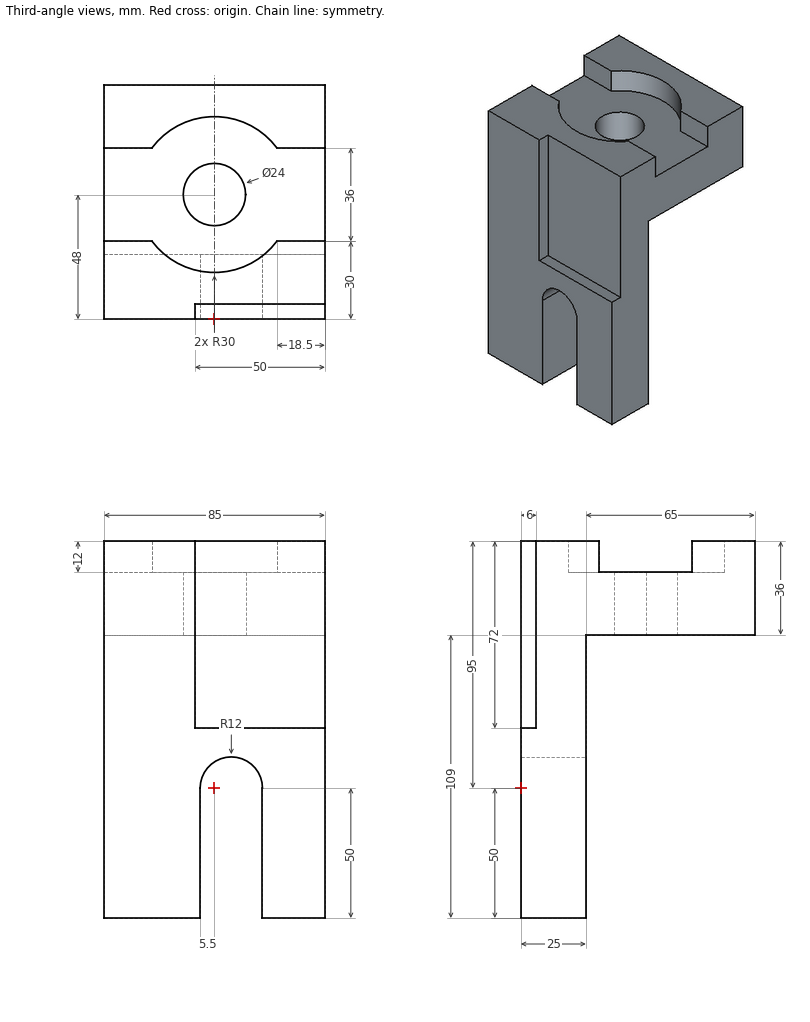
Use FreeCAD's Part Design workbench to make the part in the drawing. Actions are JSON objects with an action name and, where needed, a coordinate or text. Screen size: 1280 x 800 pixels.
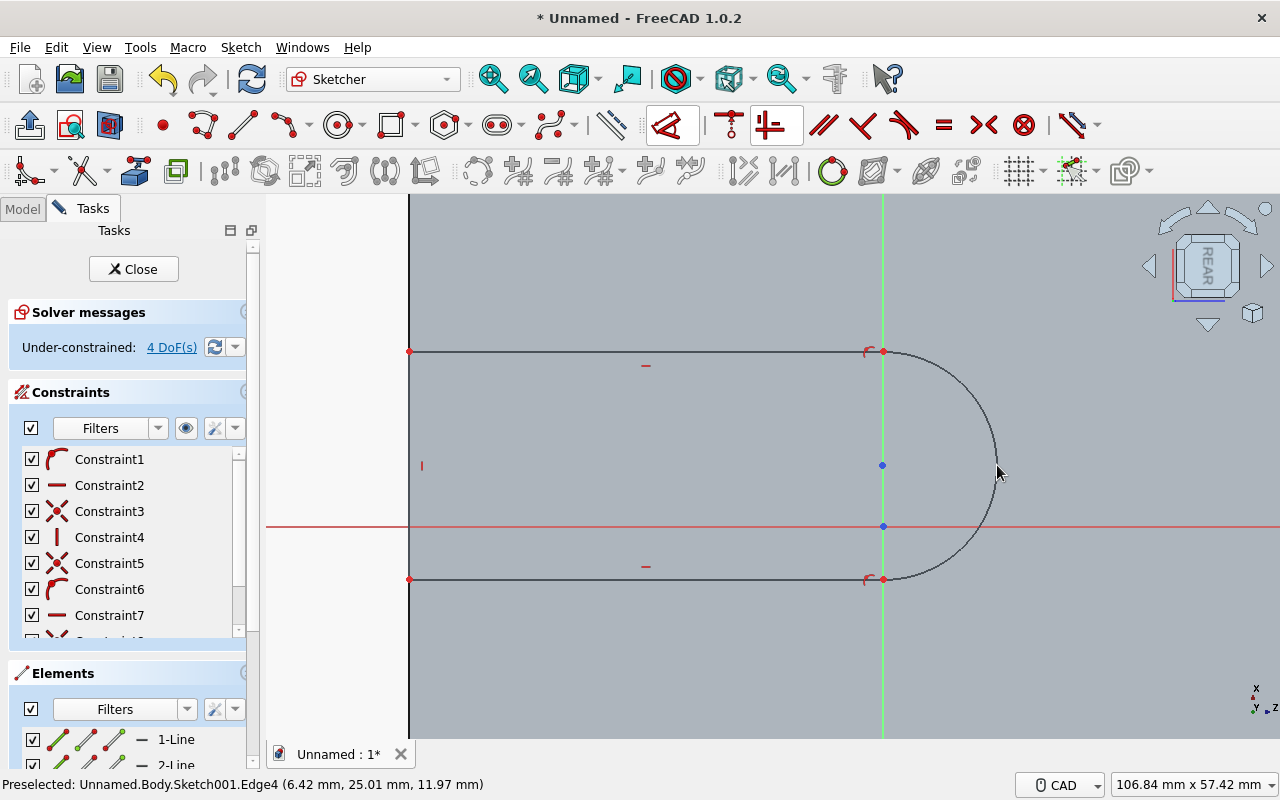
{"action": "left_click", "coordinate": [741, 352]}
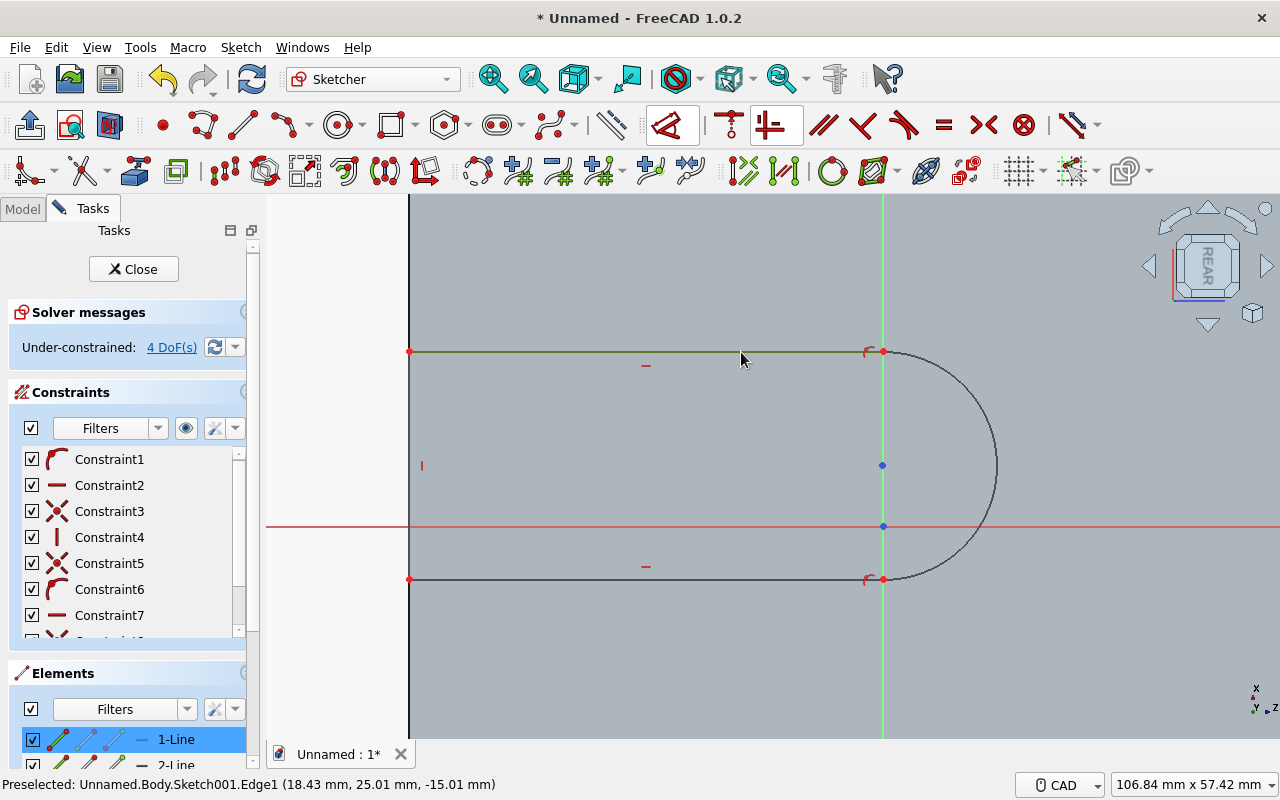
{"action": "left_click", "coordinate": [975, 399]}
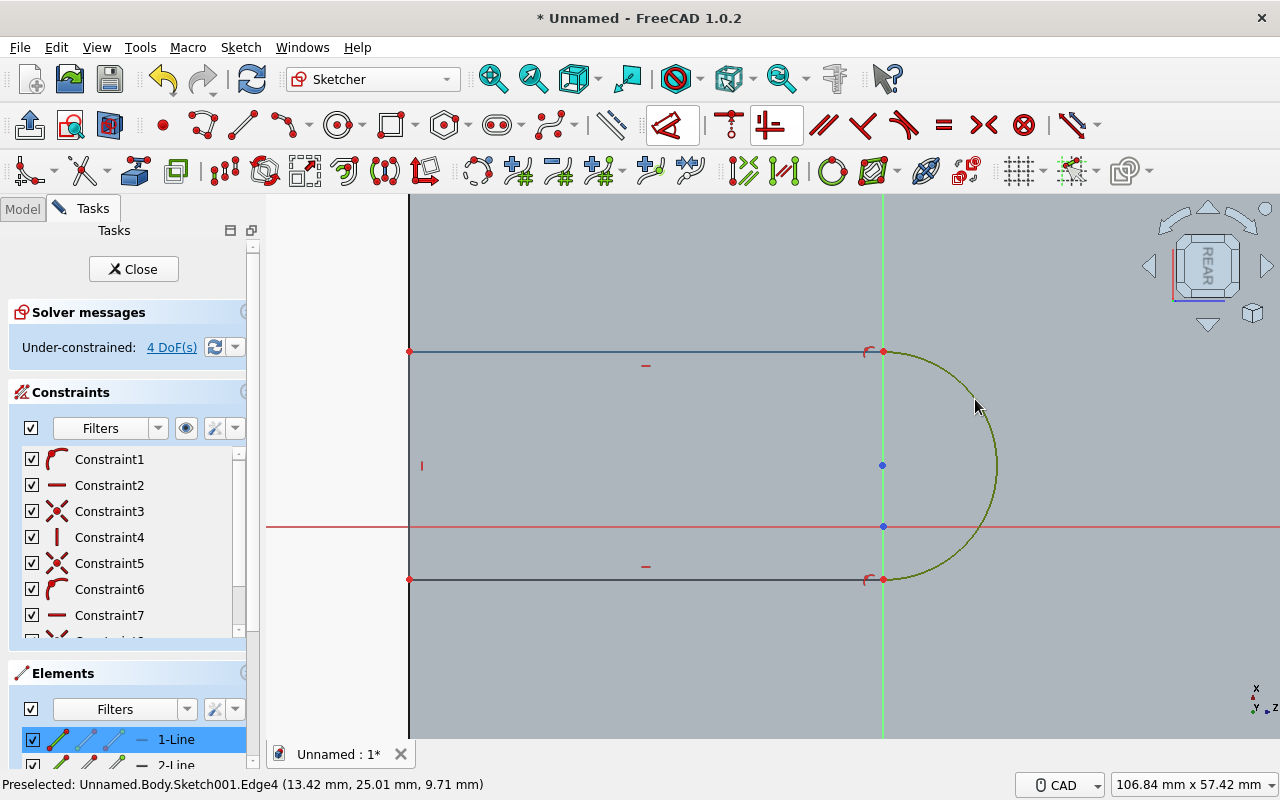
{"action": "left_click", "coordinate": [904, 126]}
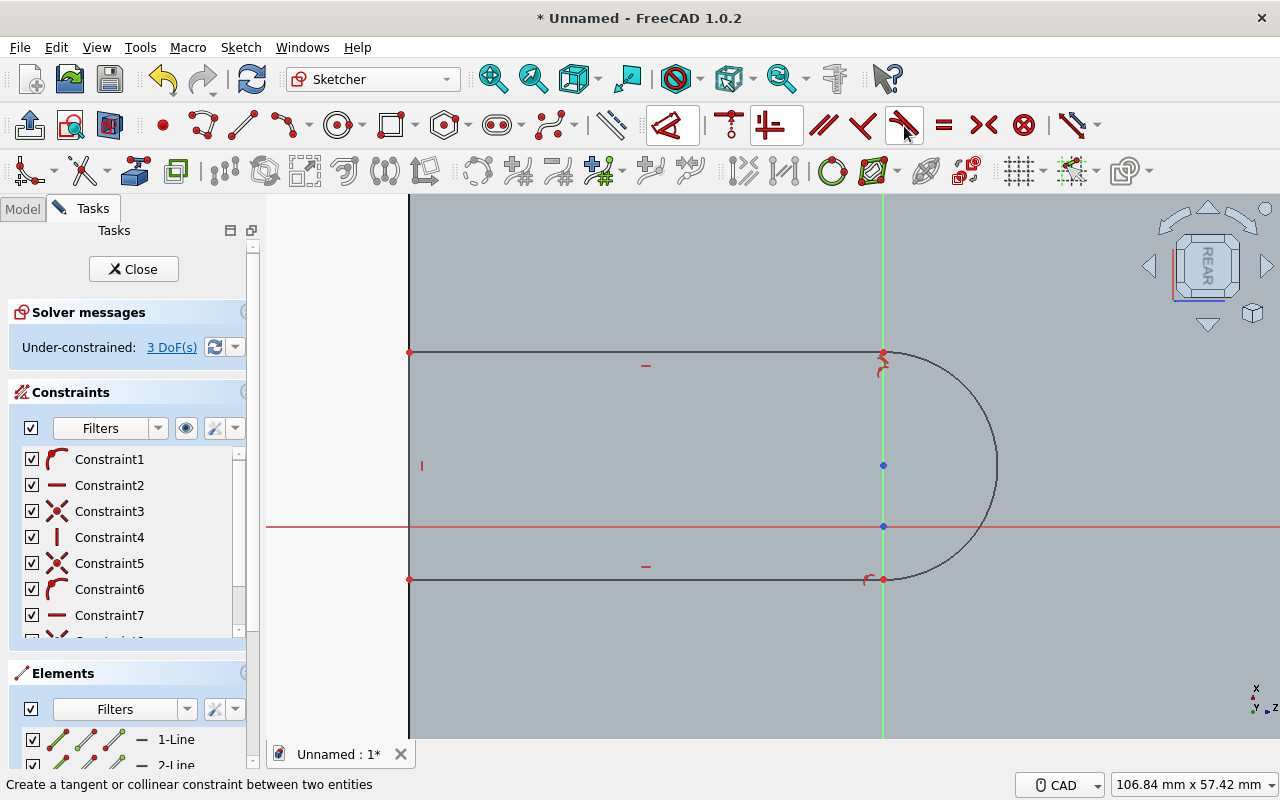
{"action": "left_click", "coordinate": [976, 399]}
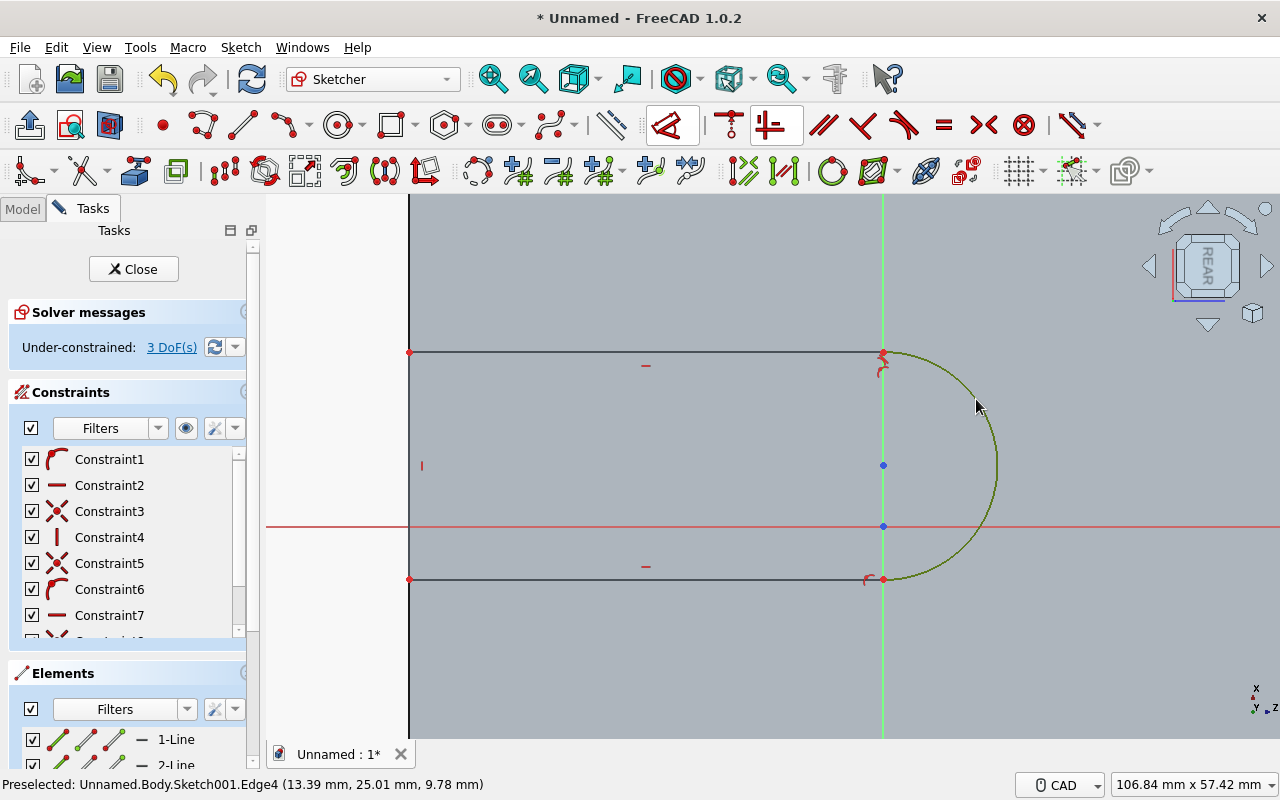
{"action": "left_click", "coordinate": [694, 126]}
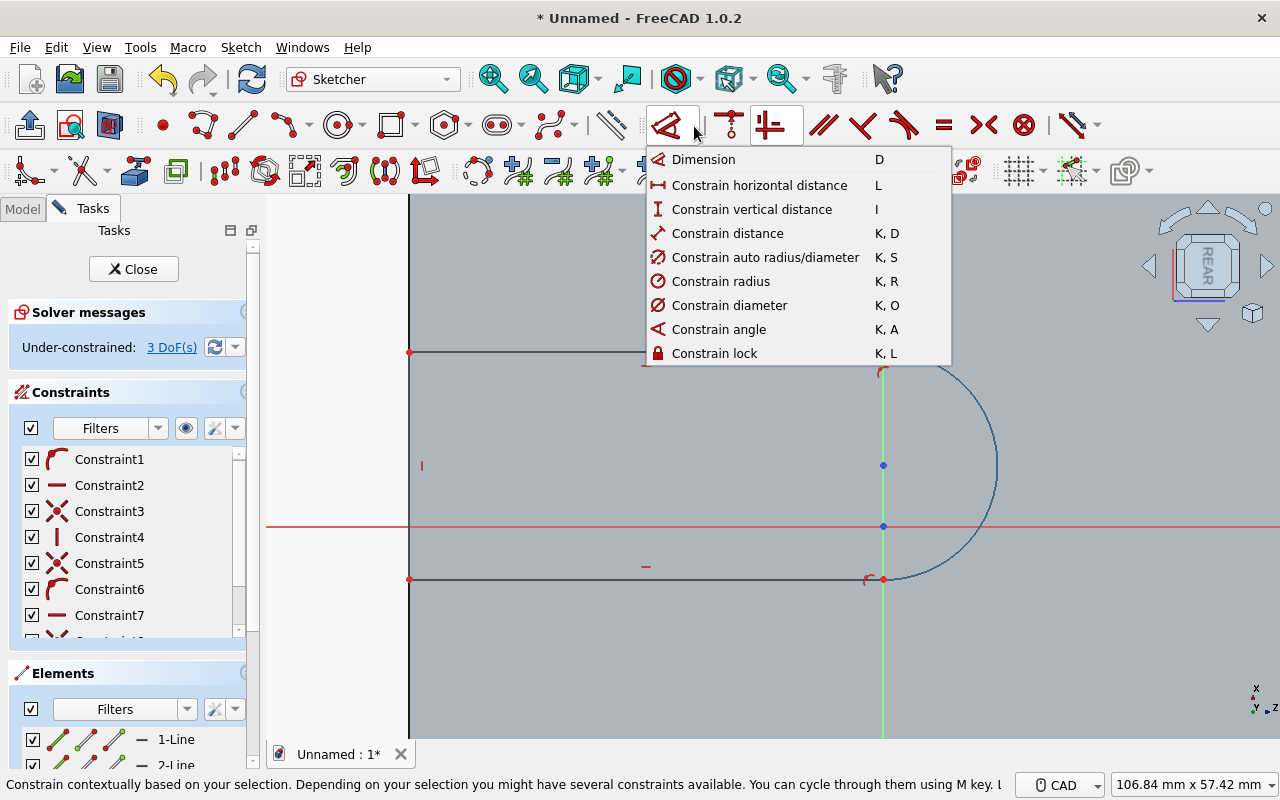
{"action": "left_click", "coordinate": [799, 281]}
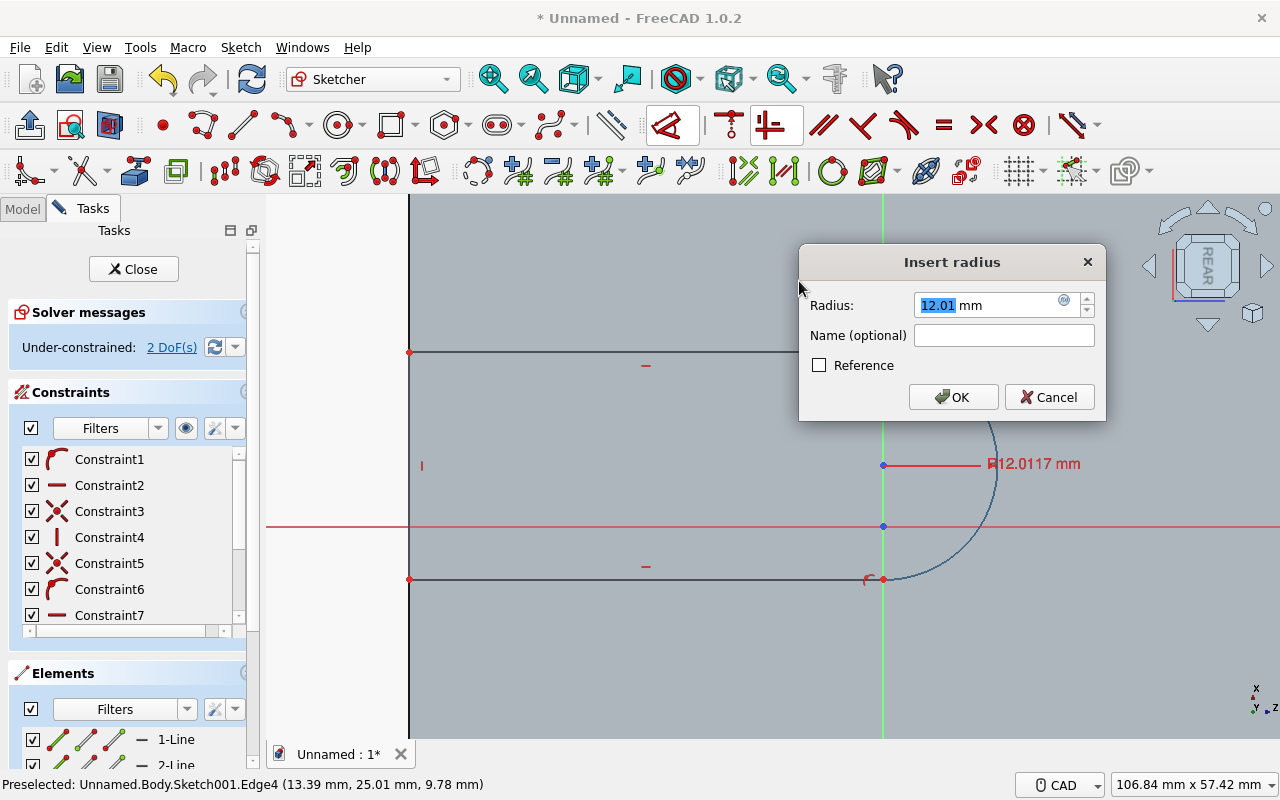
{"action": "type", "text": "12"}
{"action": "key", "text": "Return"}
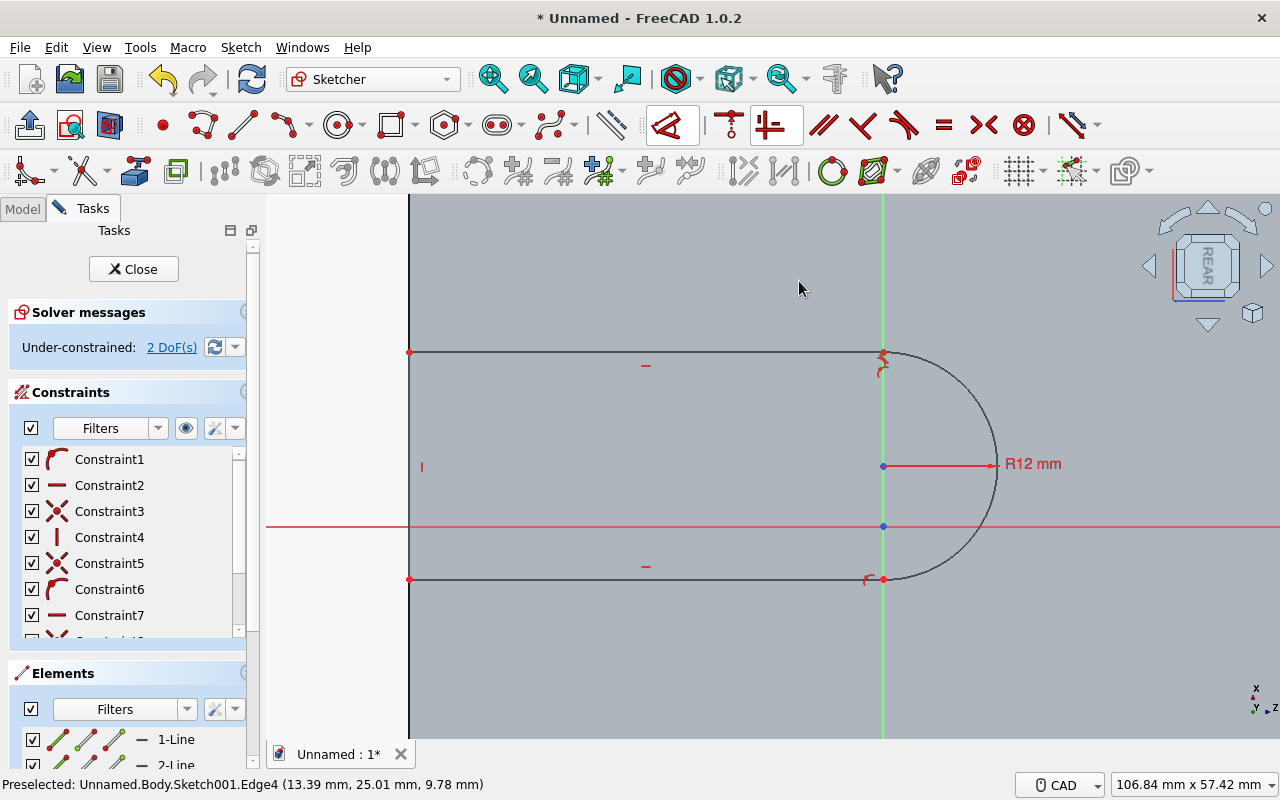
{"action": "left_click", "coordinate": [741, 352]}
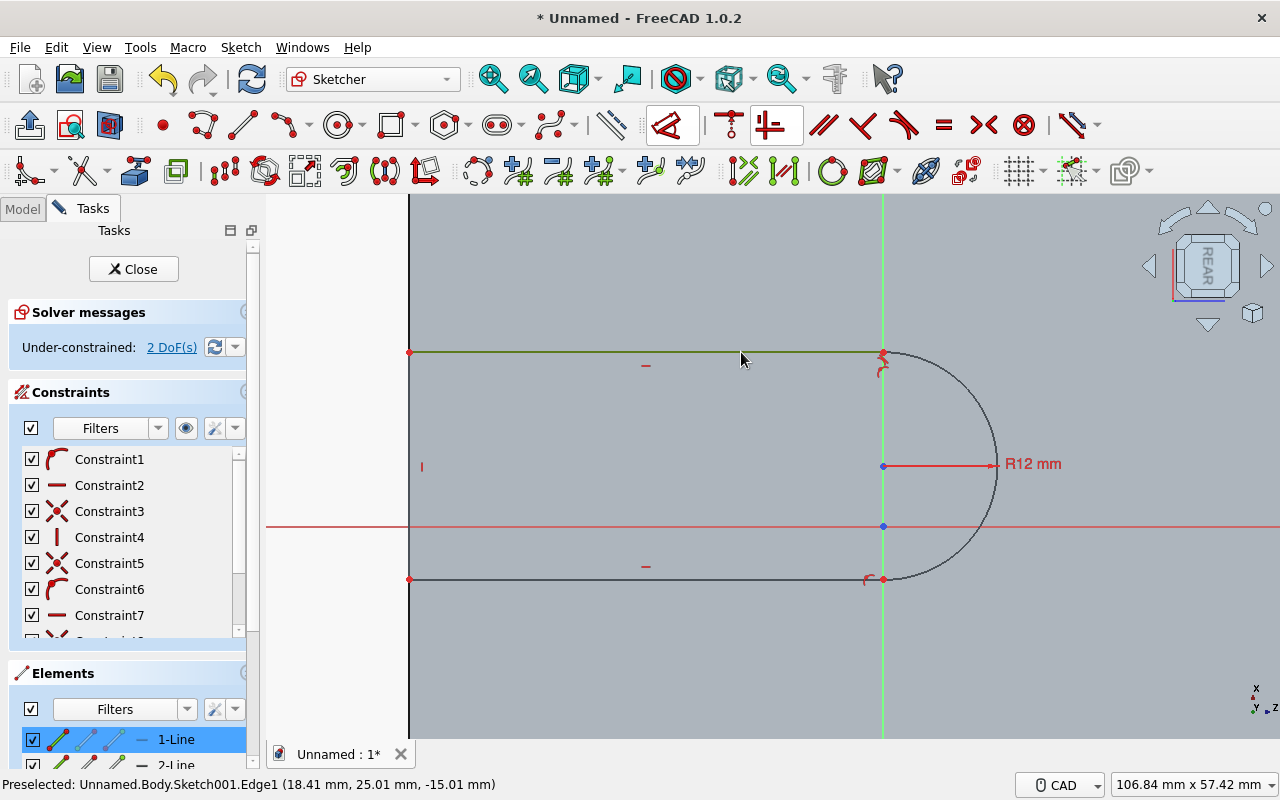
{"action": "key", "text": "l"}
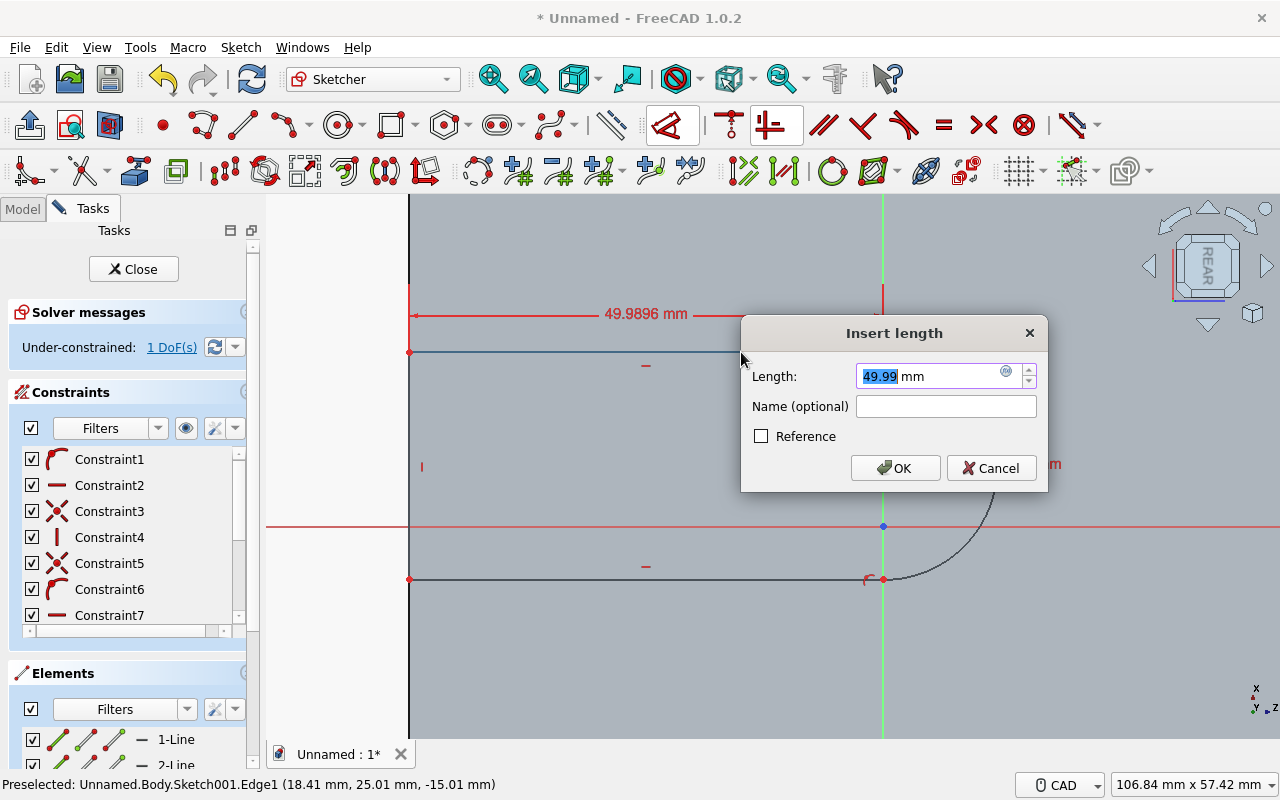
{"action": "type", "text": "50"}
{"action": "key", "text": "Return"}